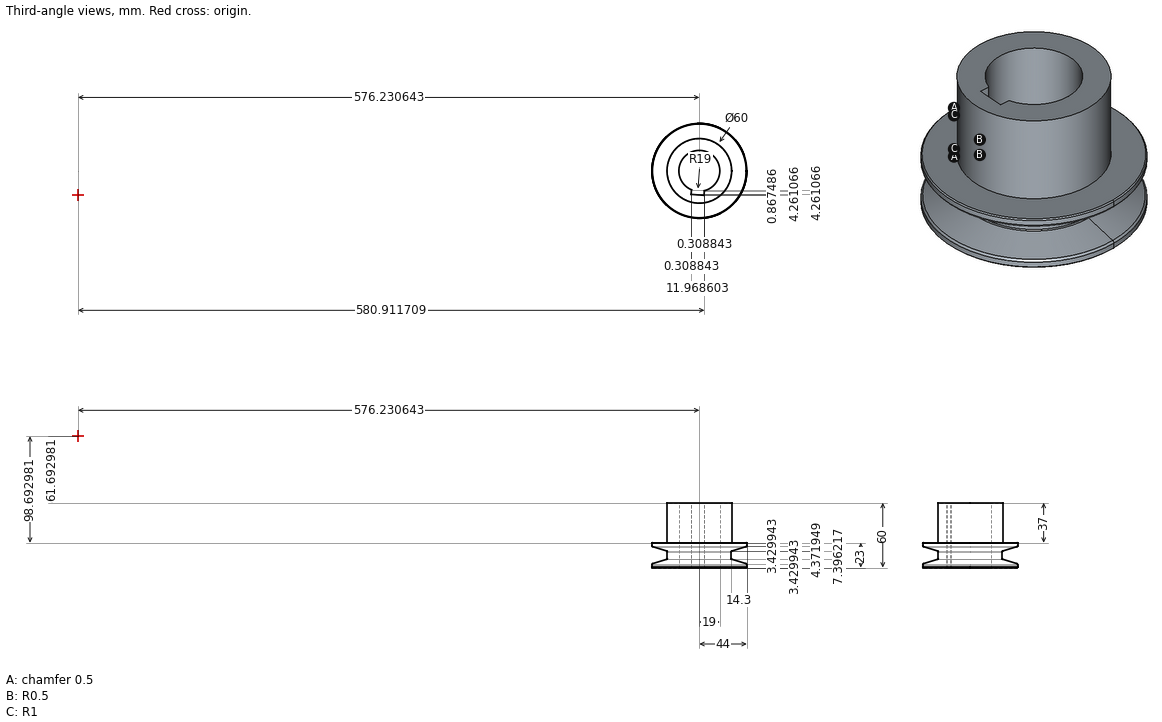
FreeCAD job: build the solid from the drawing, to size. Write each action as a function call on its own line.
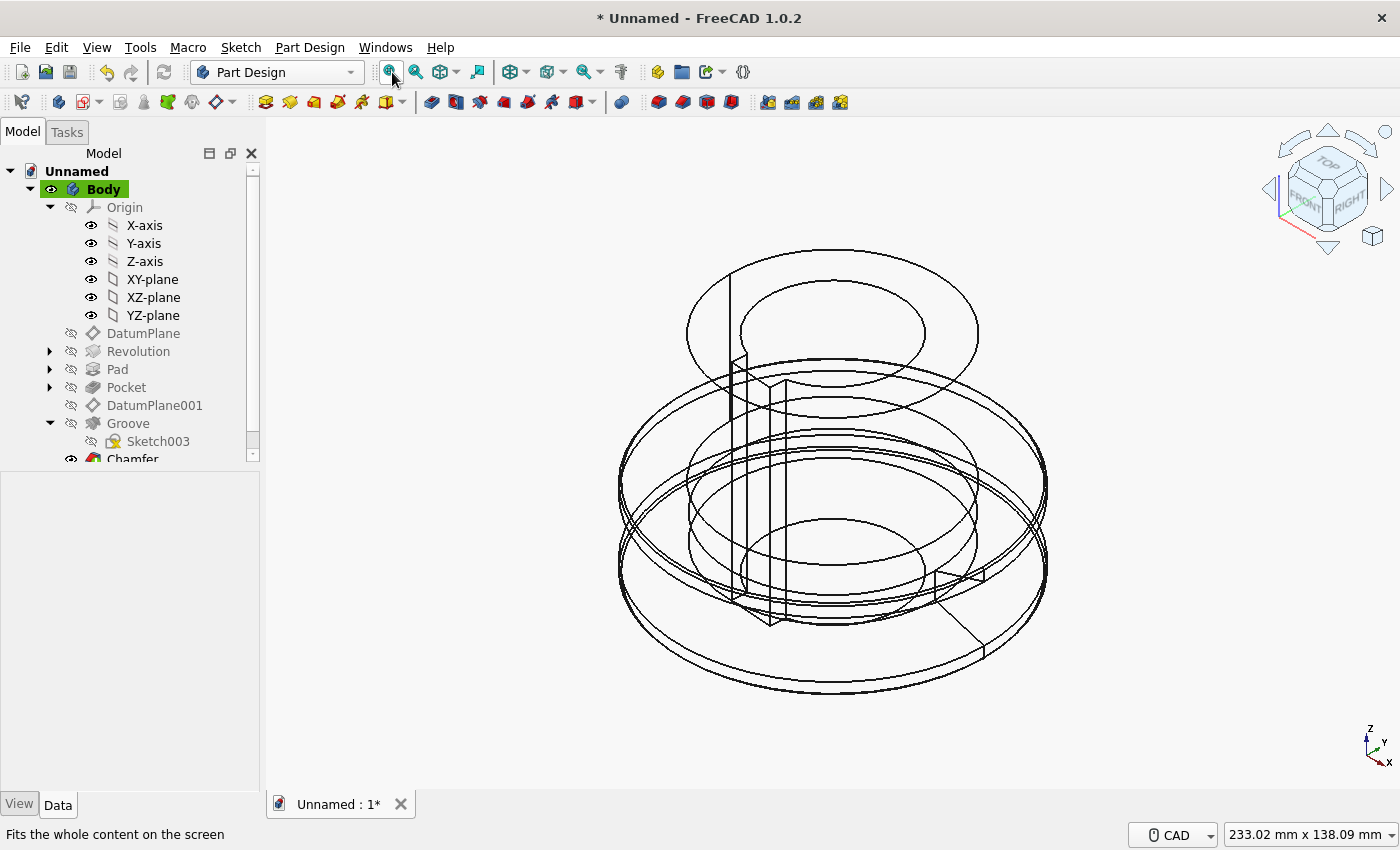
click(810, 458)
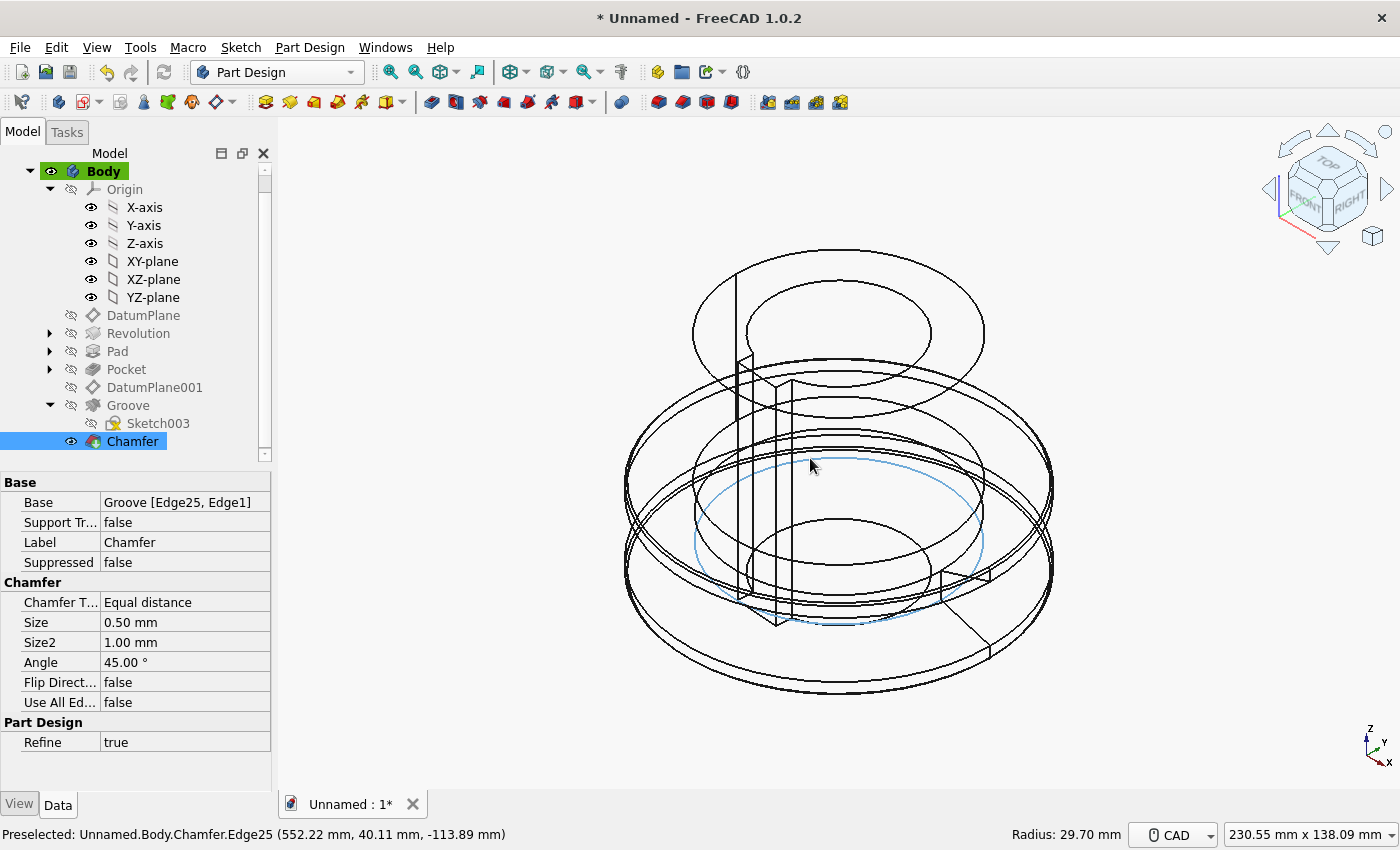
click(816, 428, ctrl)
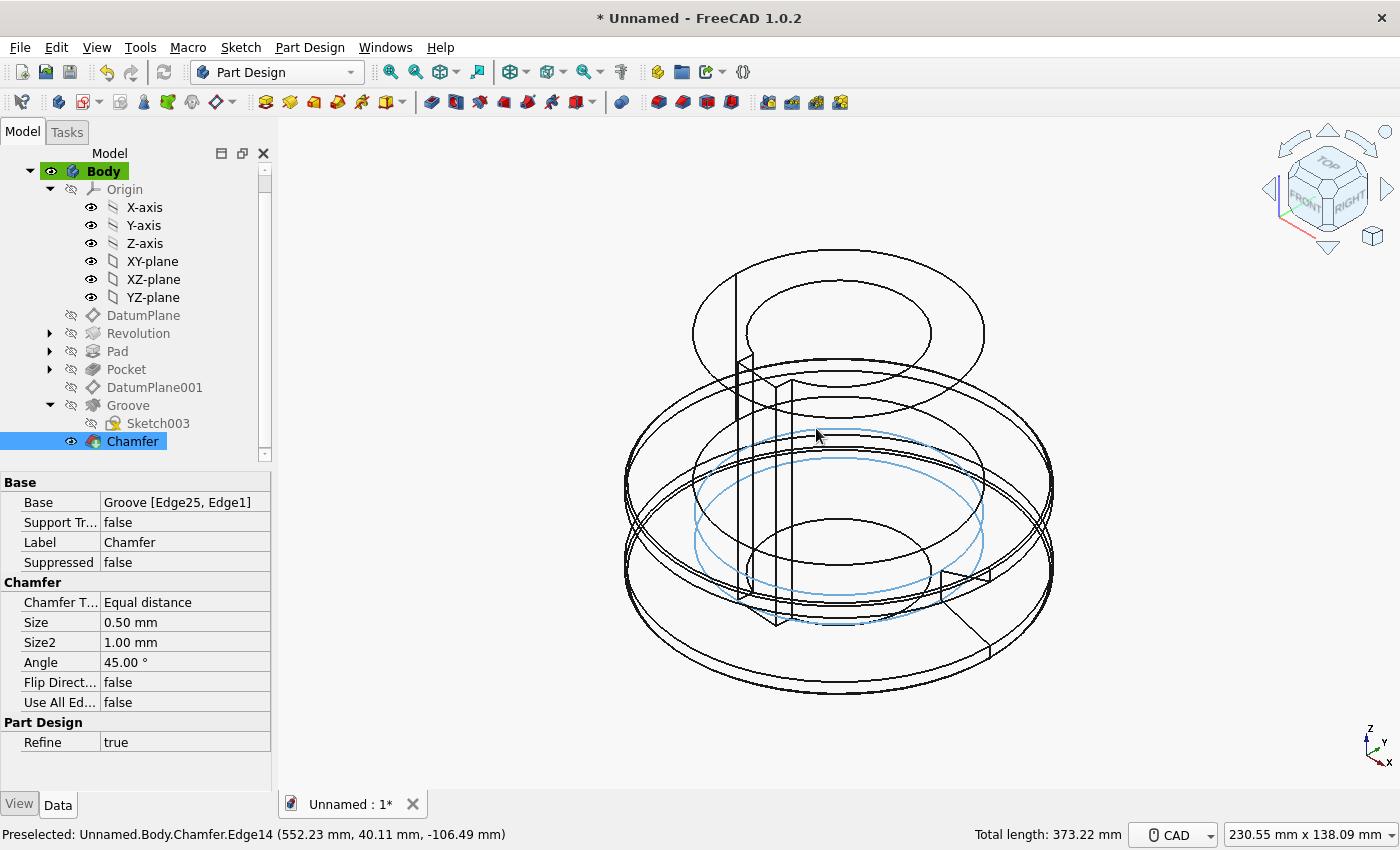
key(v)
key(1)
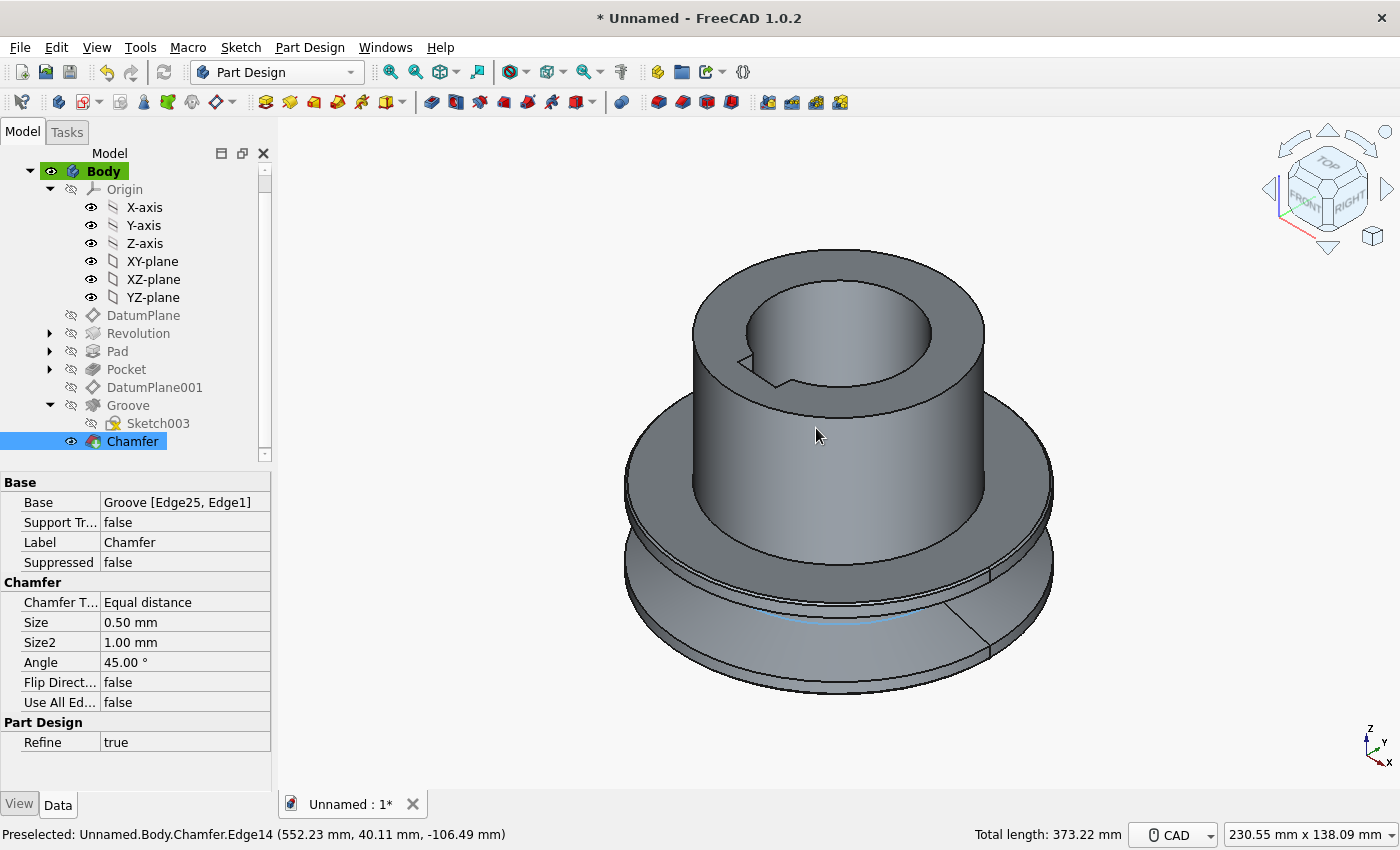
click(660, 102)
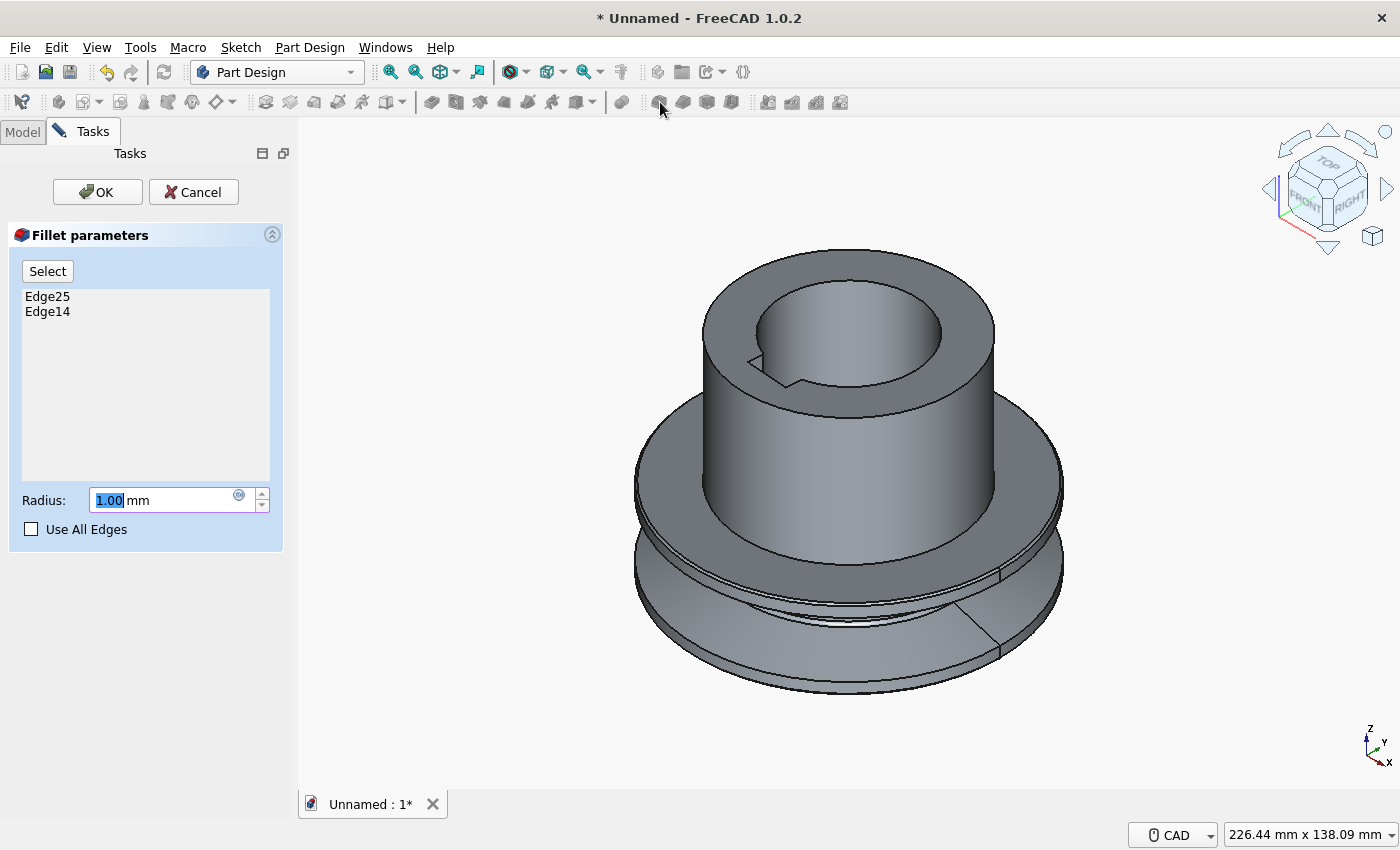
text(0.5)
key(Tab)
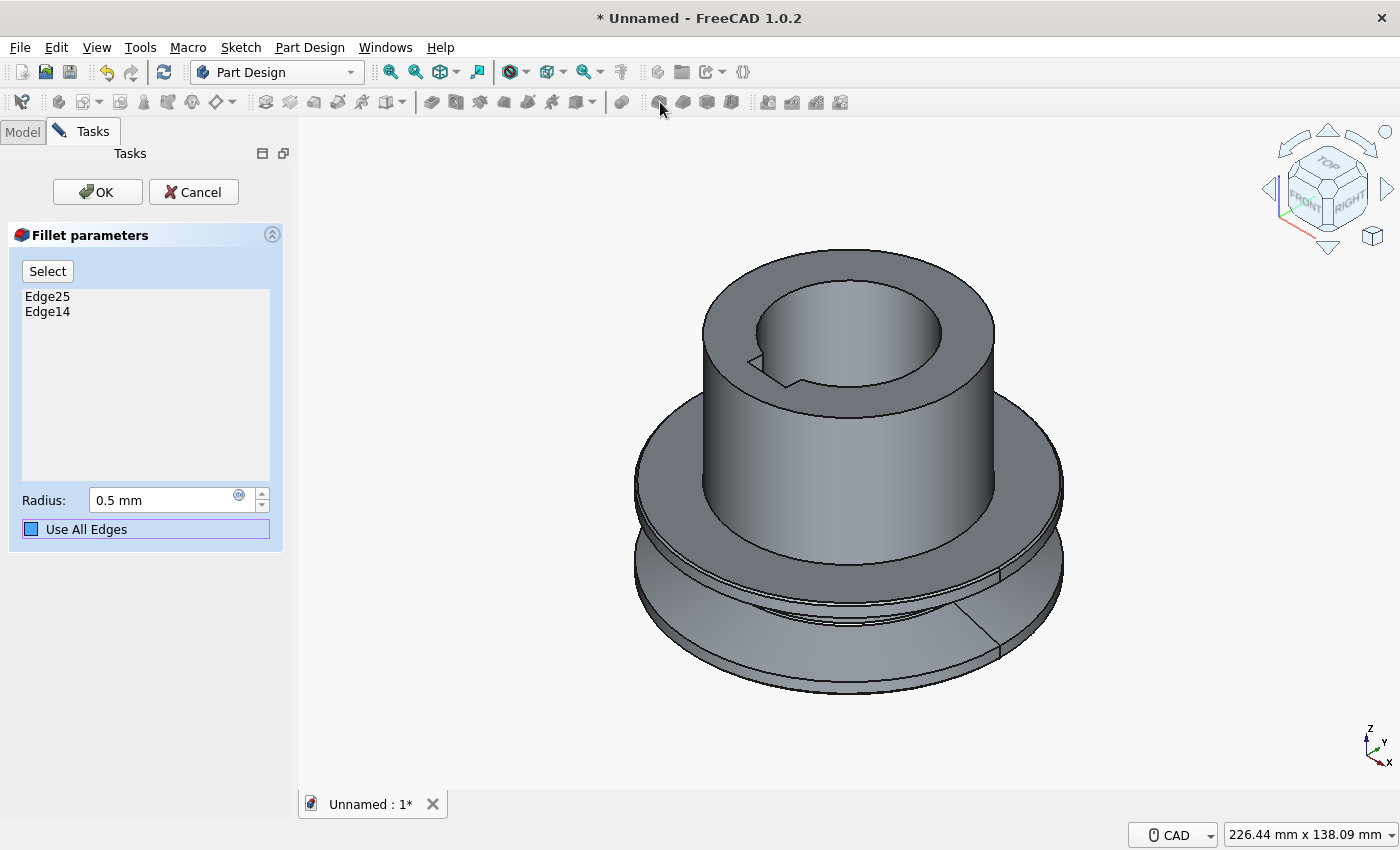
click(98, 192)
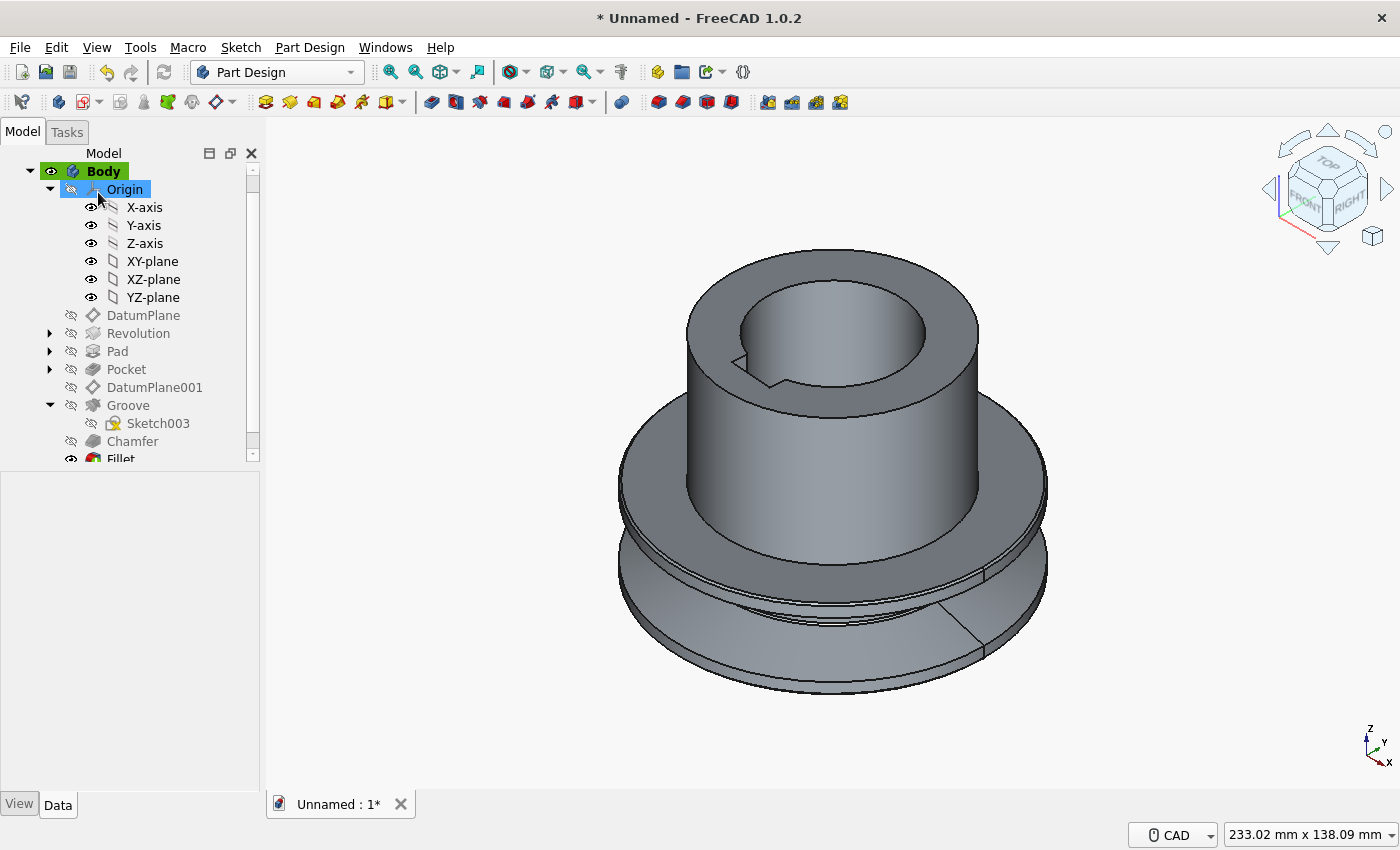
click(621, 538)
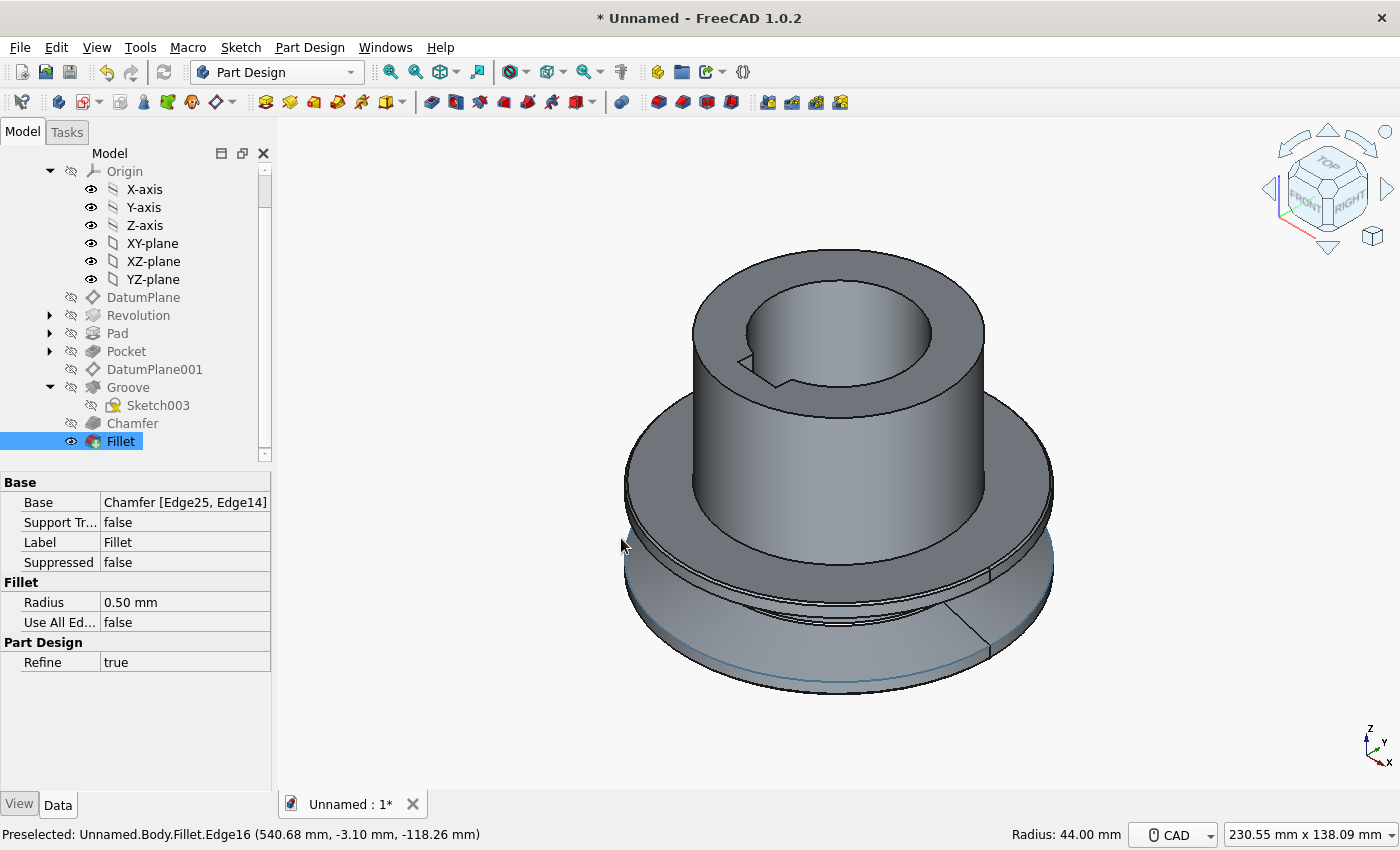
key(2)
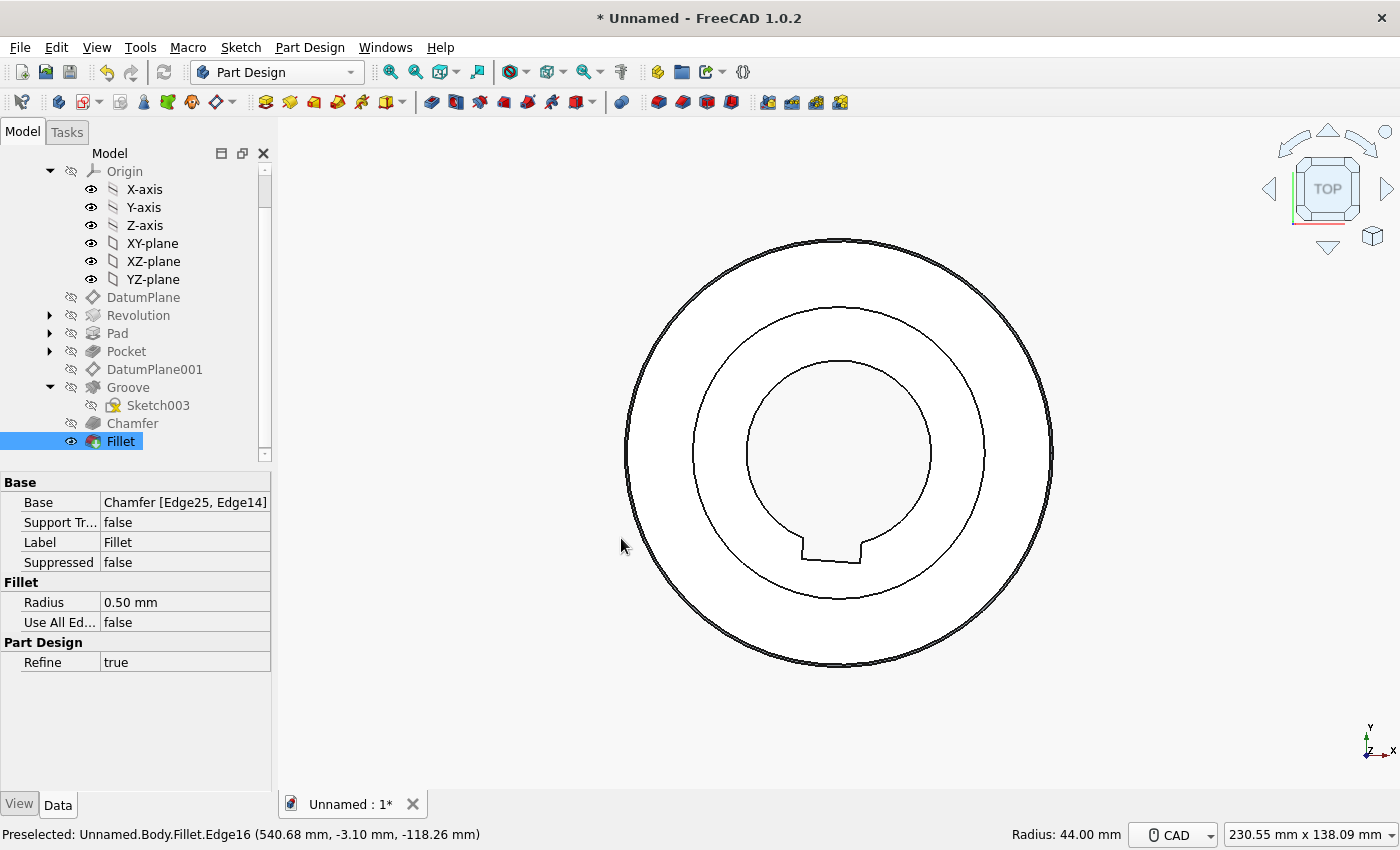
key(0)